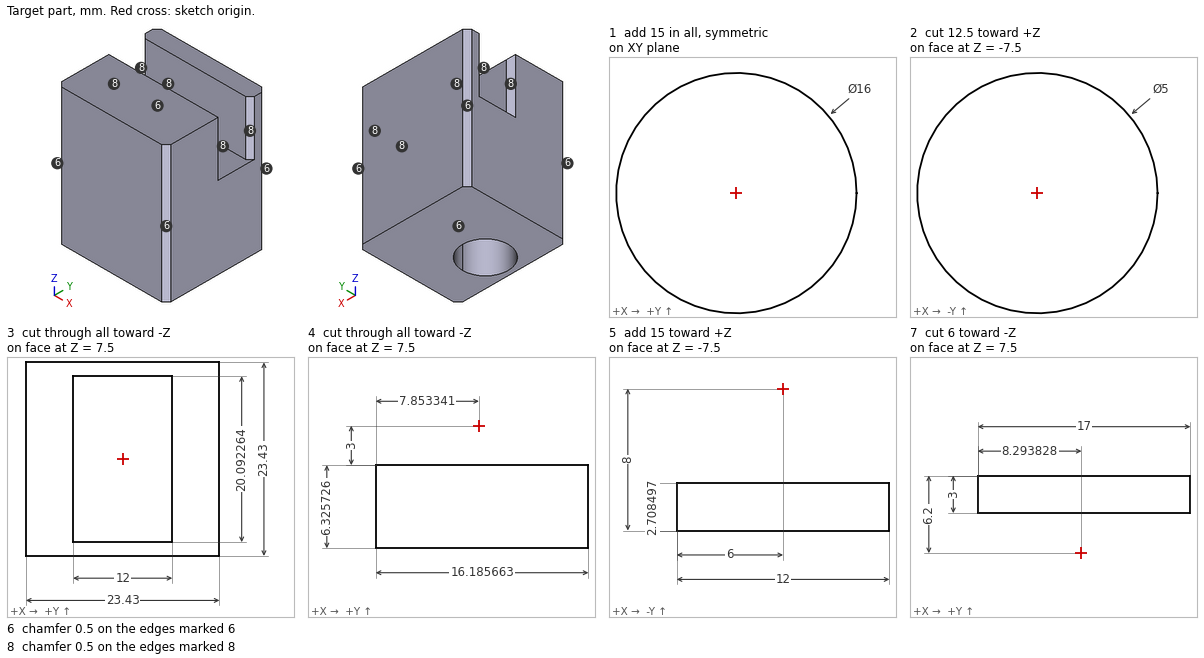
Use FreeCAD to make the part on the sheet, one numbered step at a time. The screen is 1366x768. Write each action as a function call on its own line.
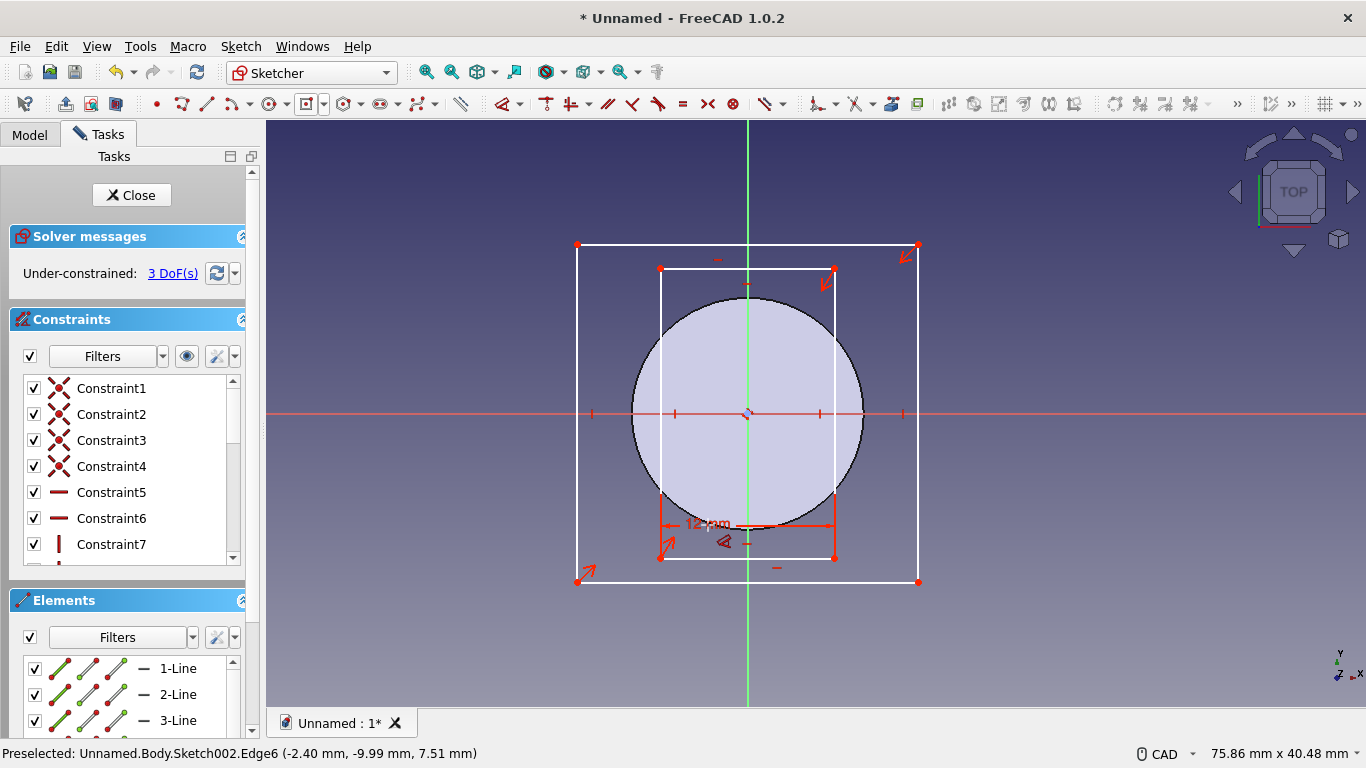
click(680, 583)
click(669, 617)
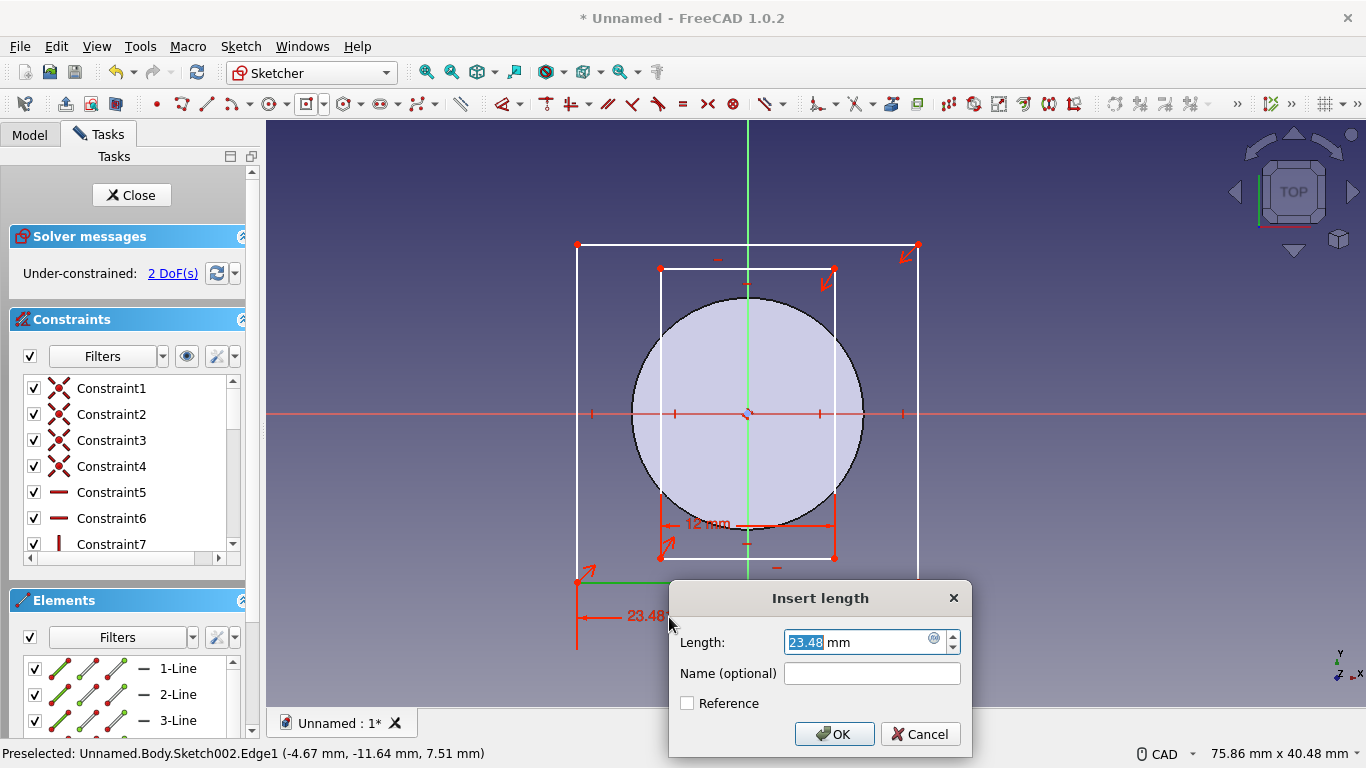
text(23.43)
key(Return)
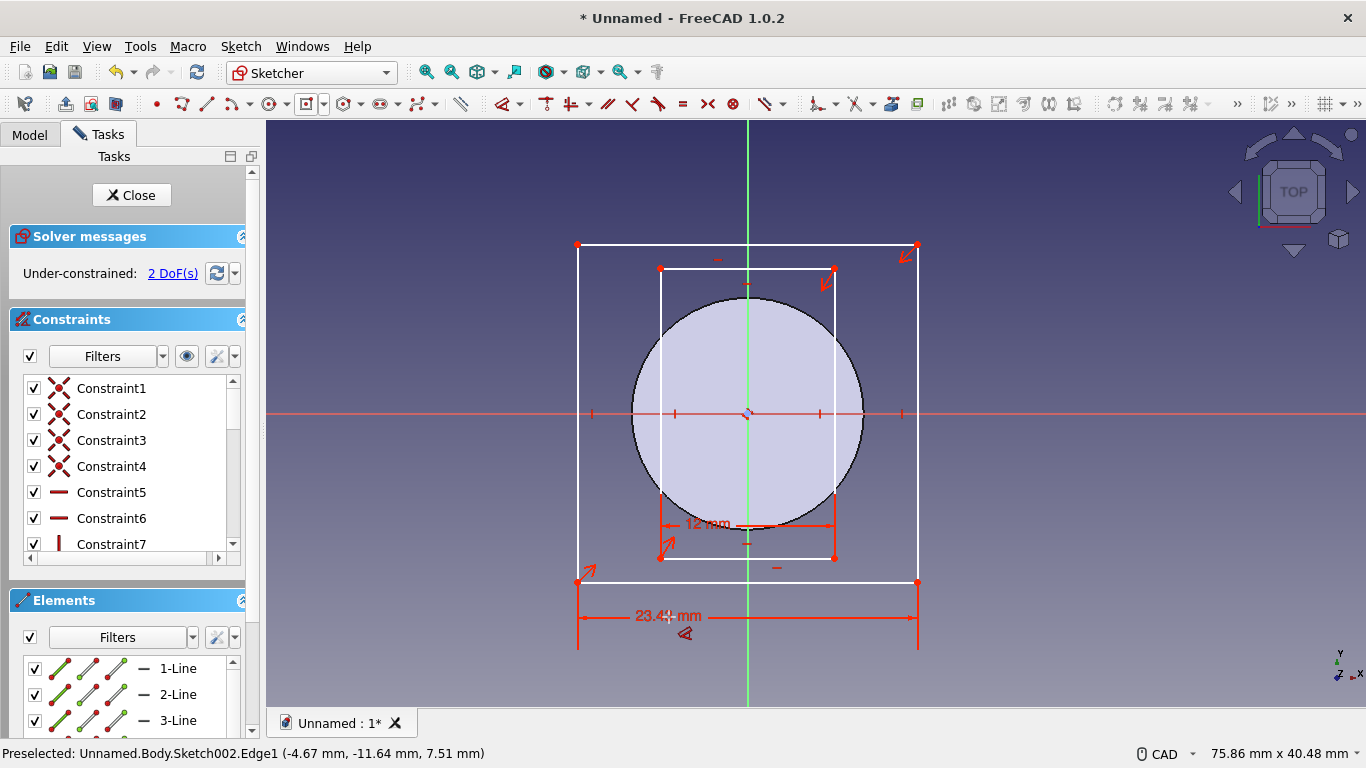
click(918, 481)
click(952, 336)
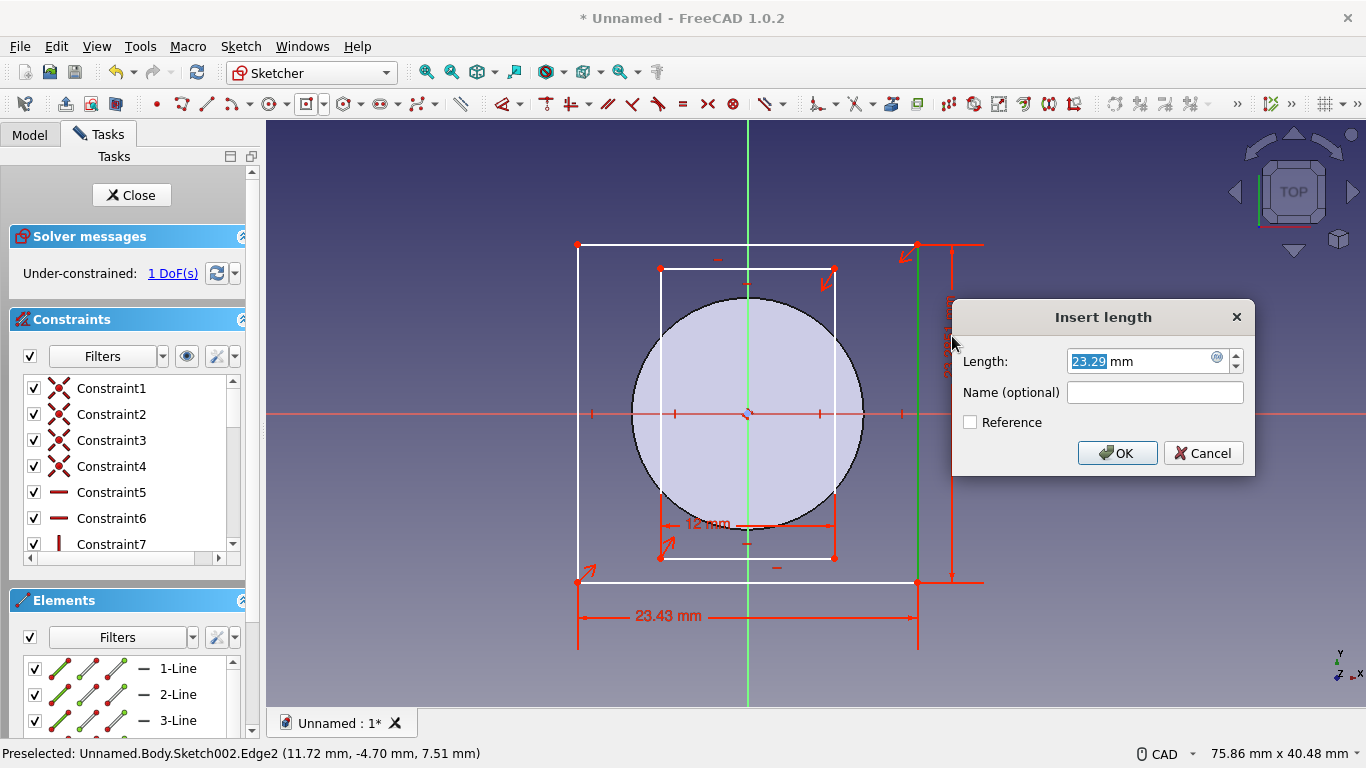
text(23.43)
key(Return)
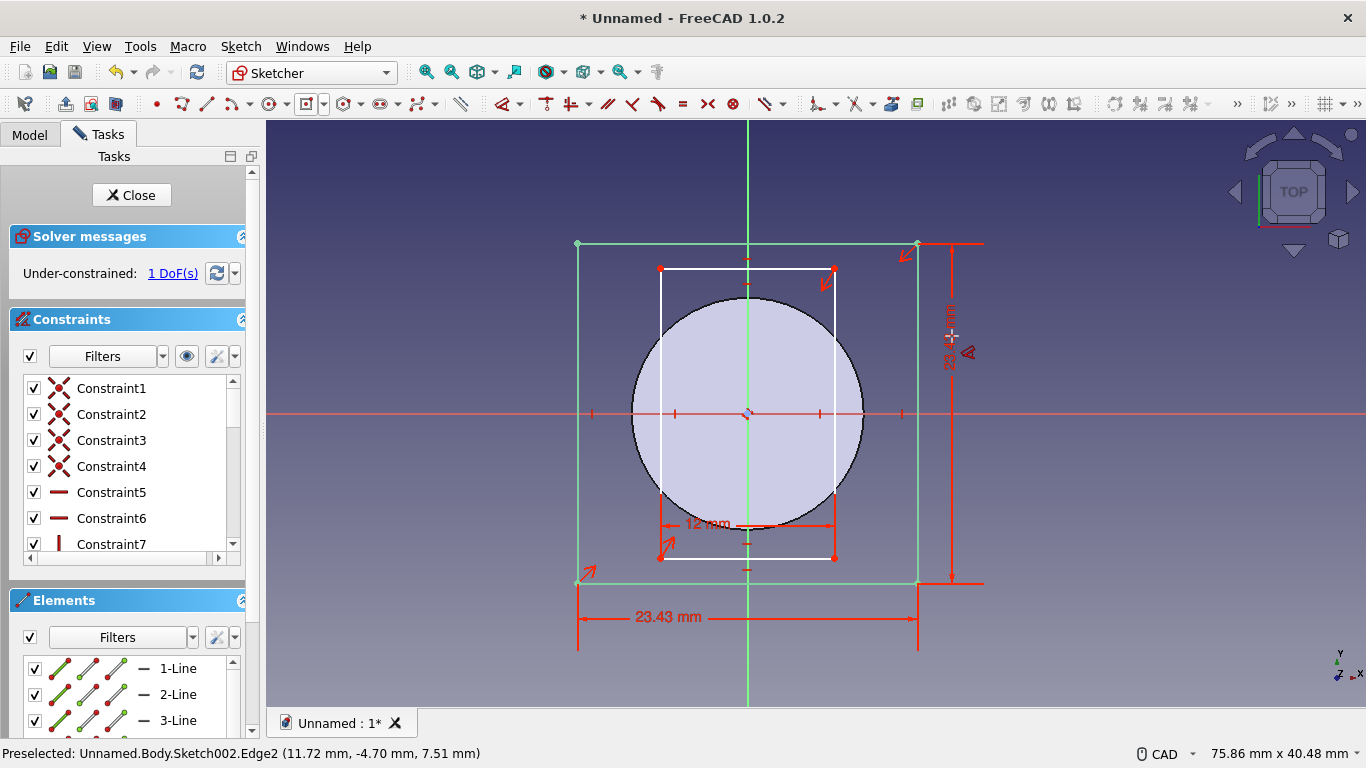
click(835, 472)
click(869, 347)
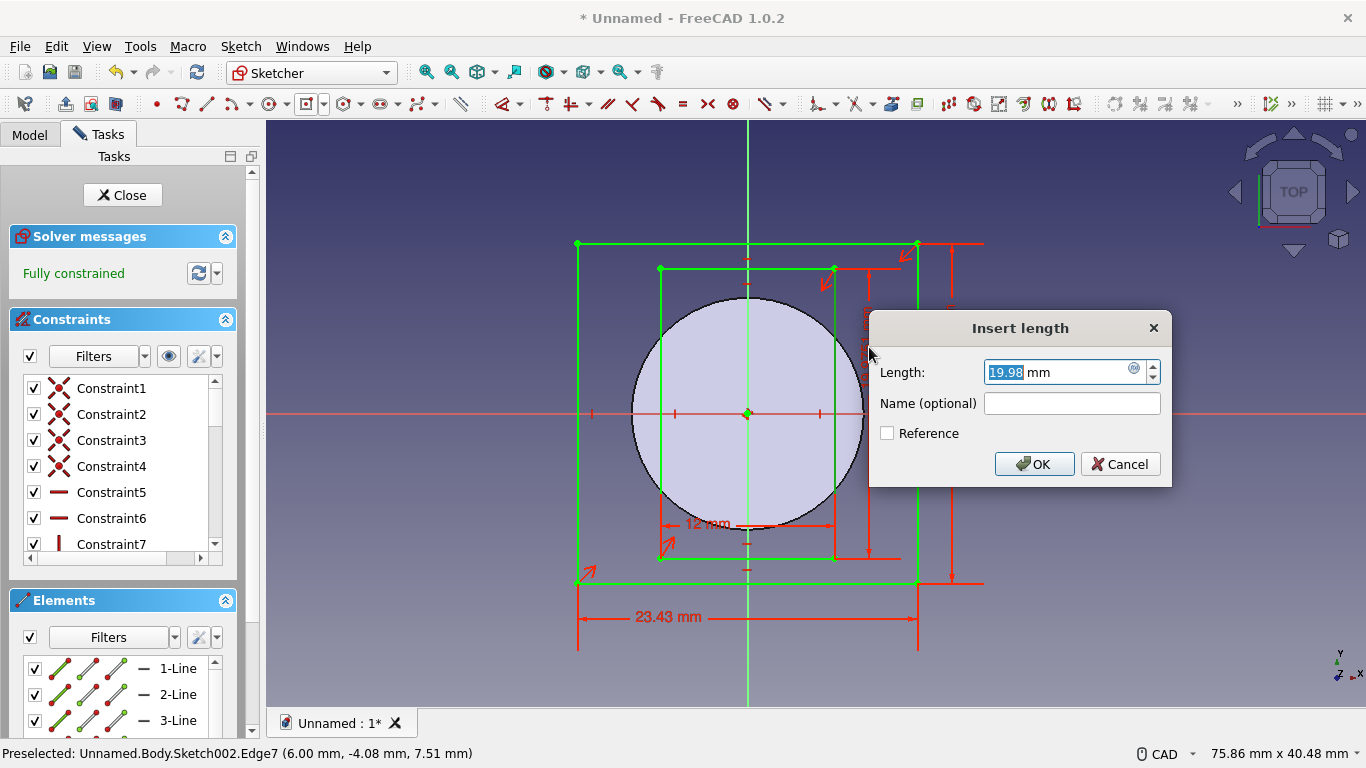
text(20.092264)
key(Return)
key(Escape)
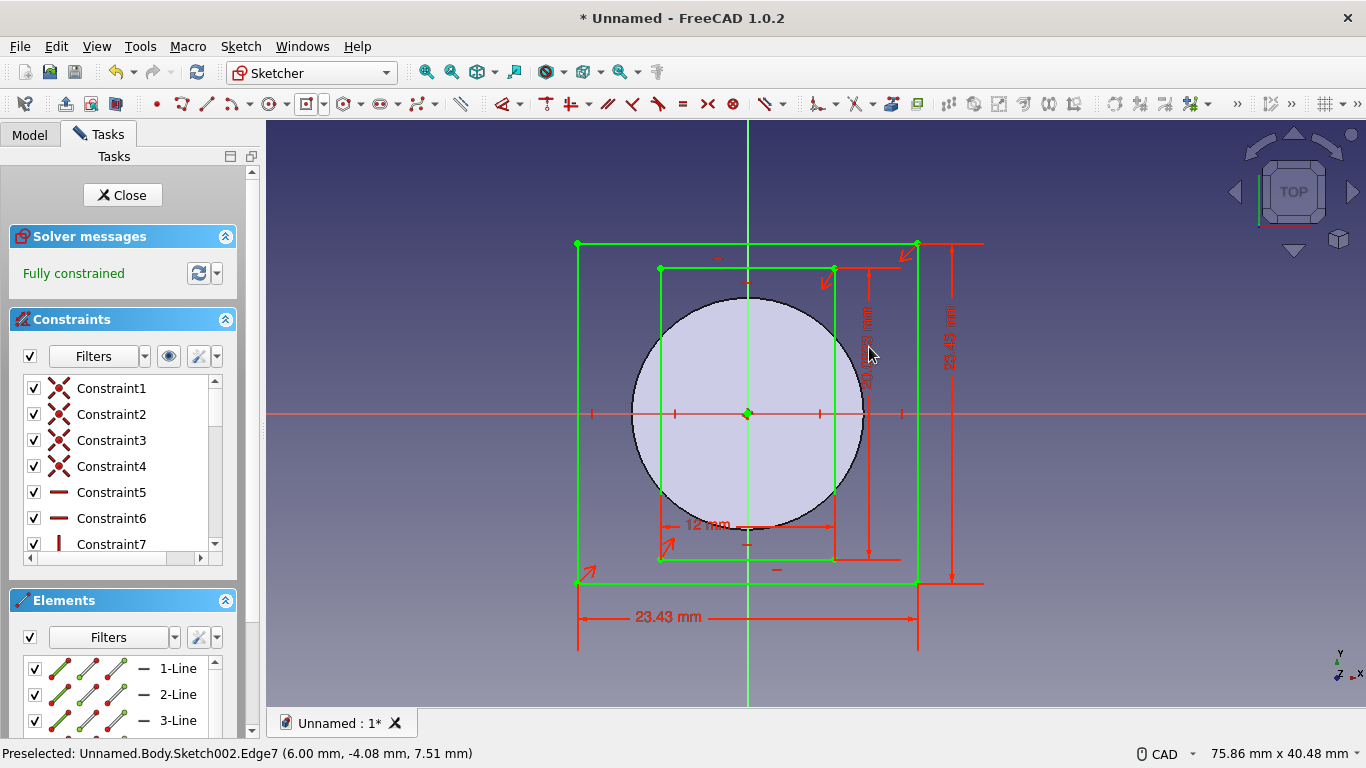
click(123, 195)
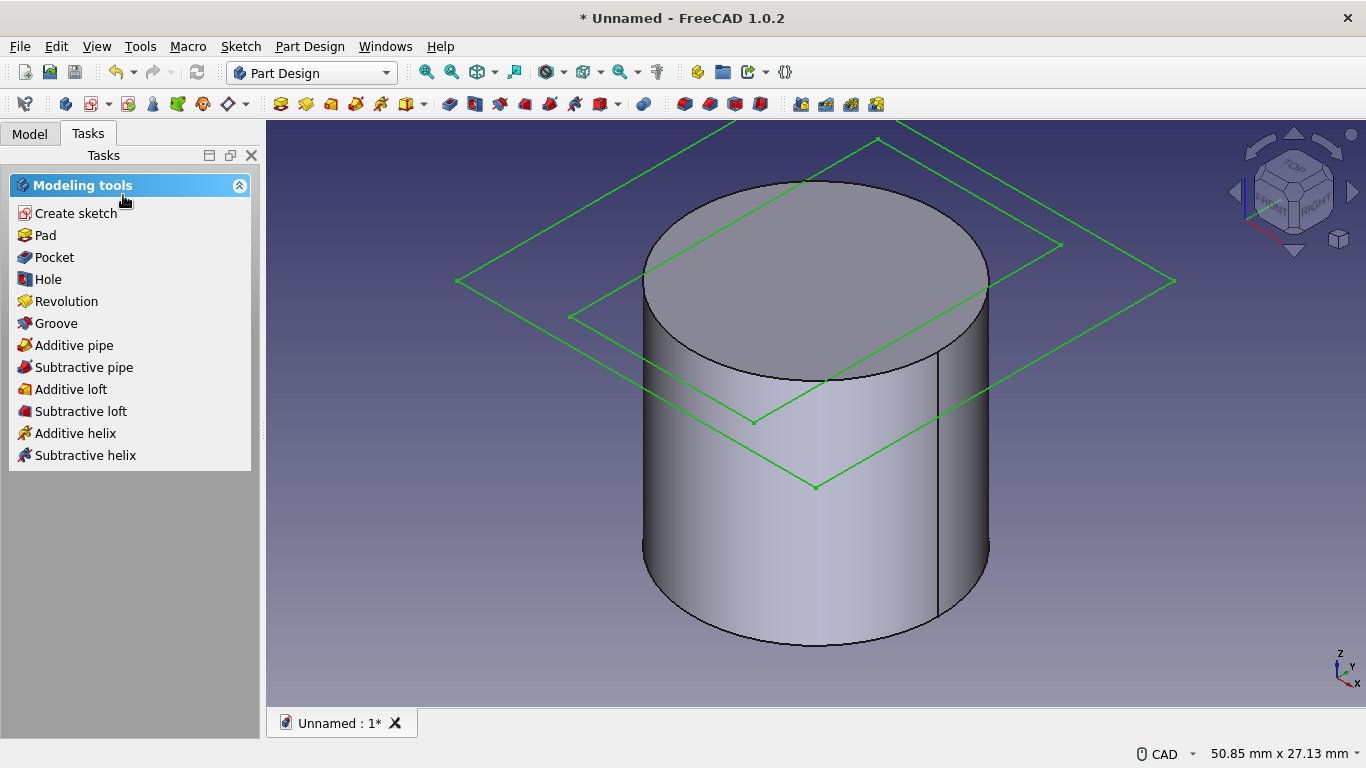
click(450, 104)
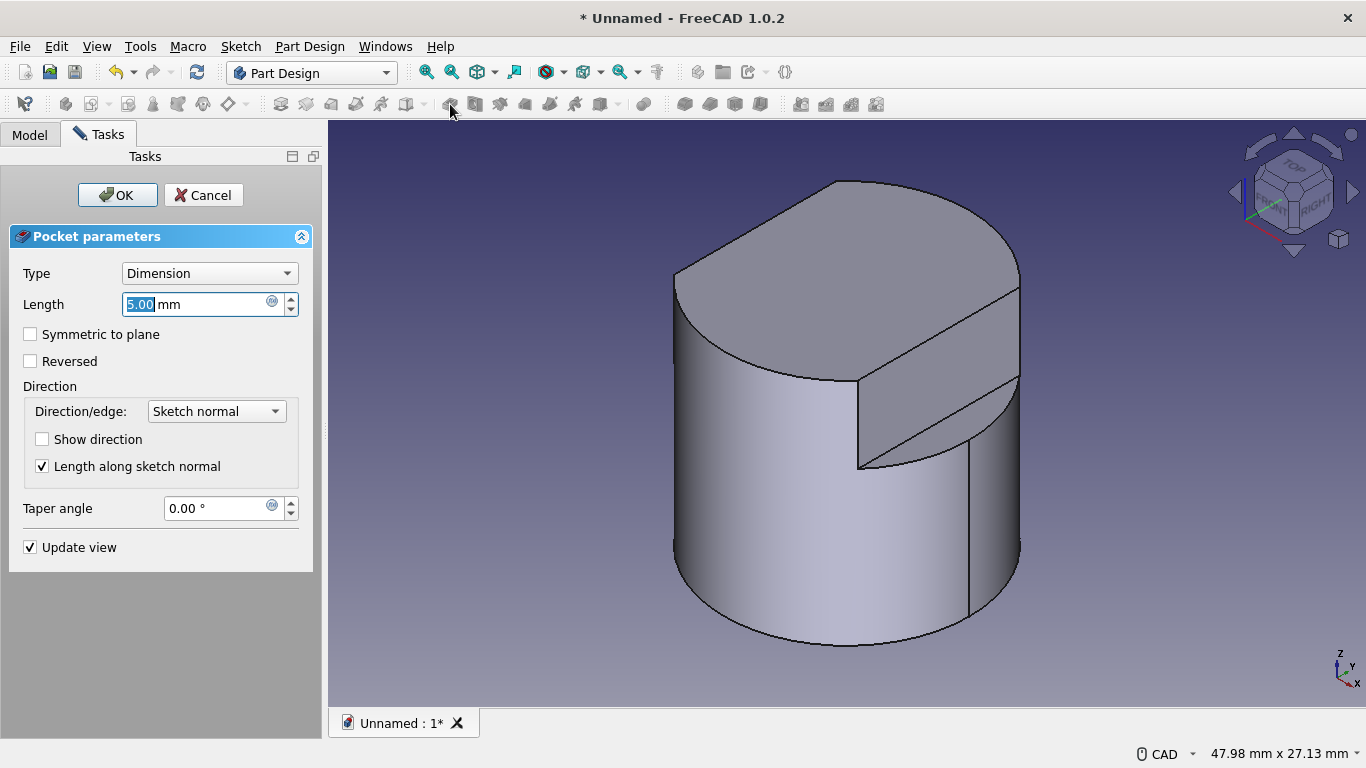
click(210, 274)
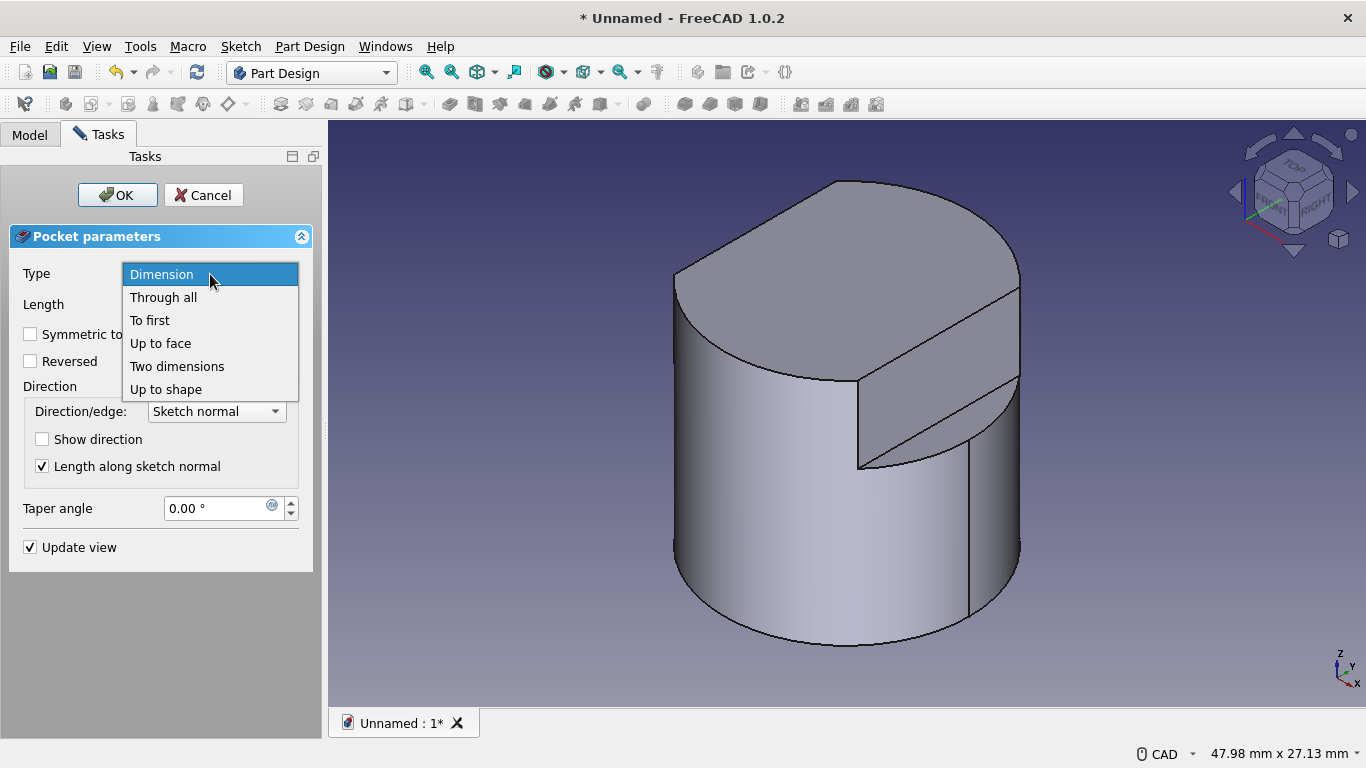
click(208, 298)